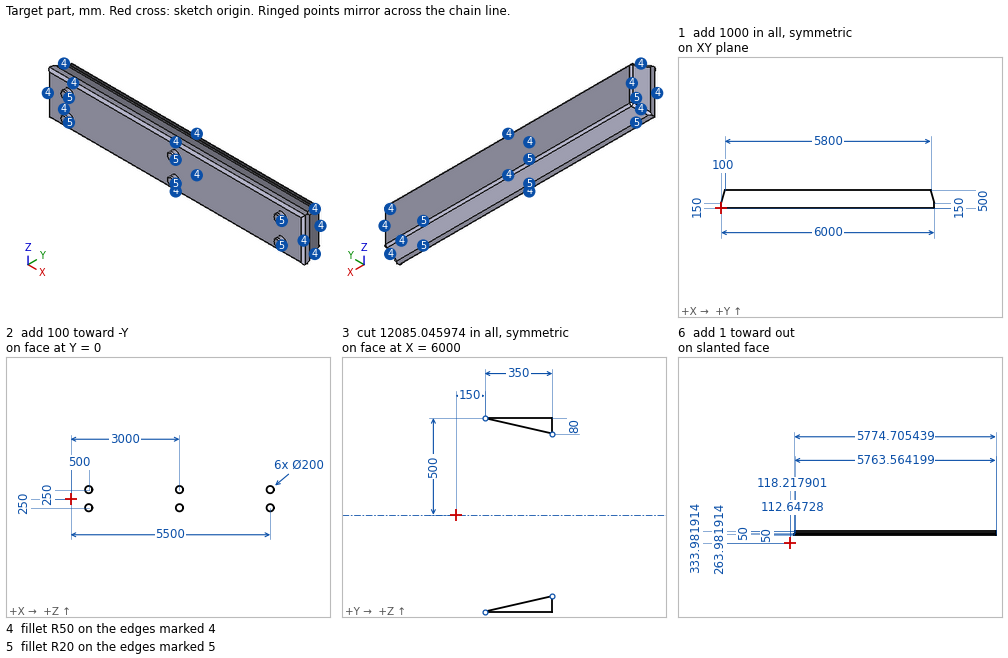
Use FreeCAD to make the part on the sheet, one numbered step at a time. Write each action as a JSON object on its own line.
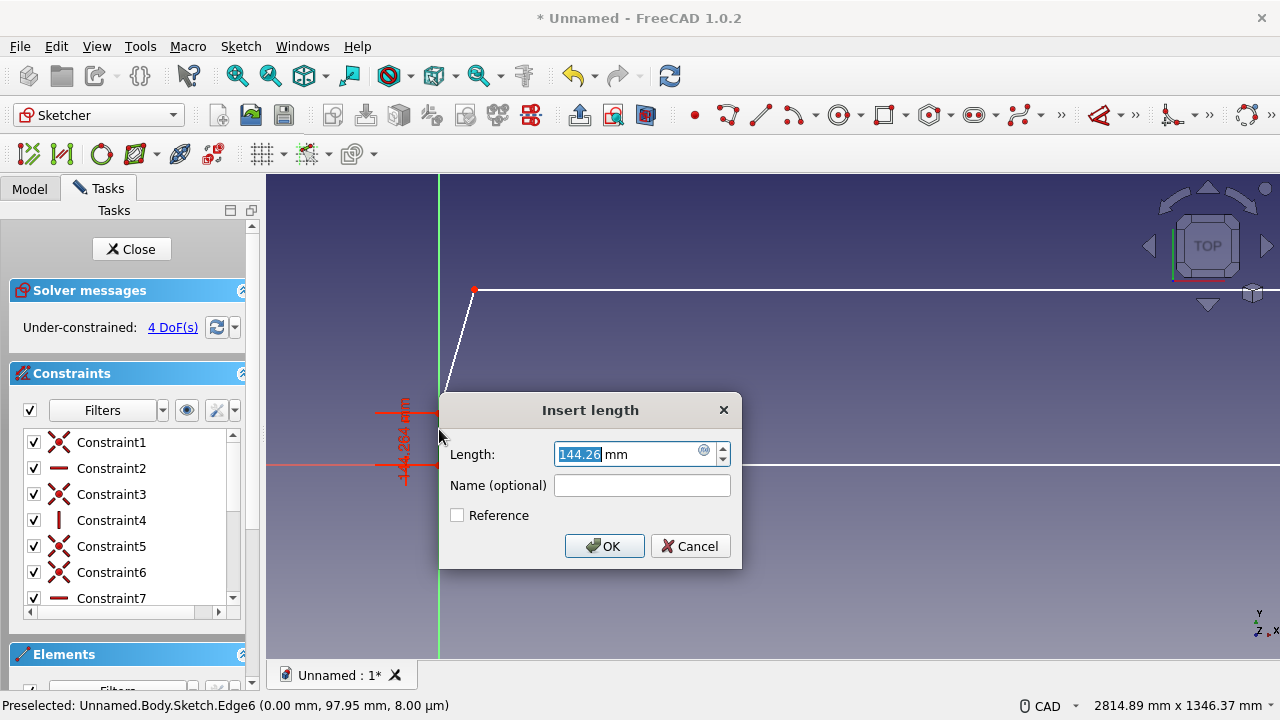
{"action": "type", "text": "150"}
{"action": "key", "text": "Return"}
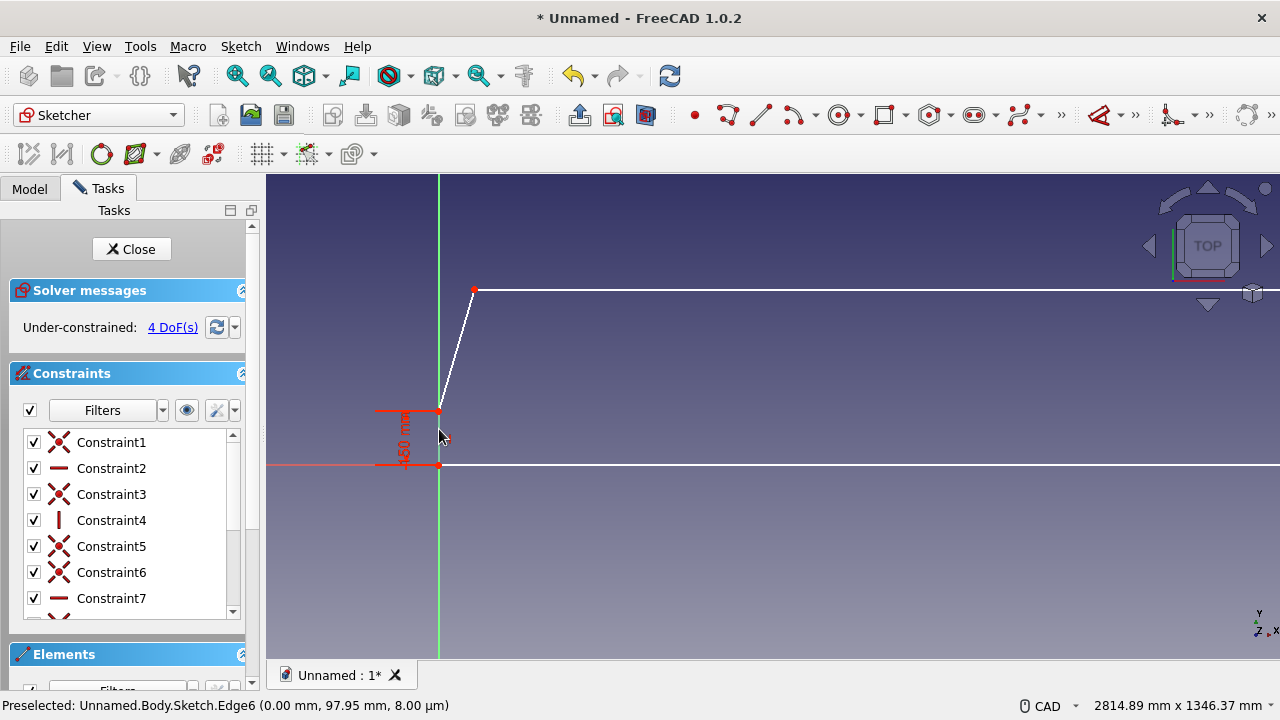
{"action": "scroll", "coordinate": [438, 430], "scroll_direction": "down", "scroll_amount": 7}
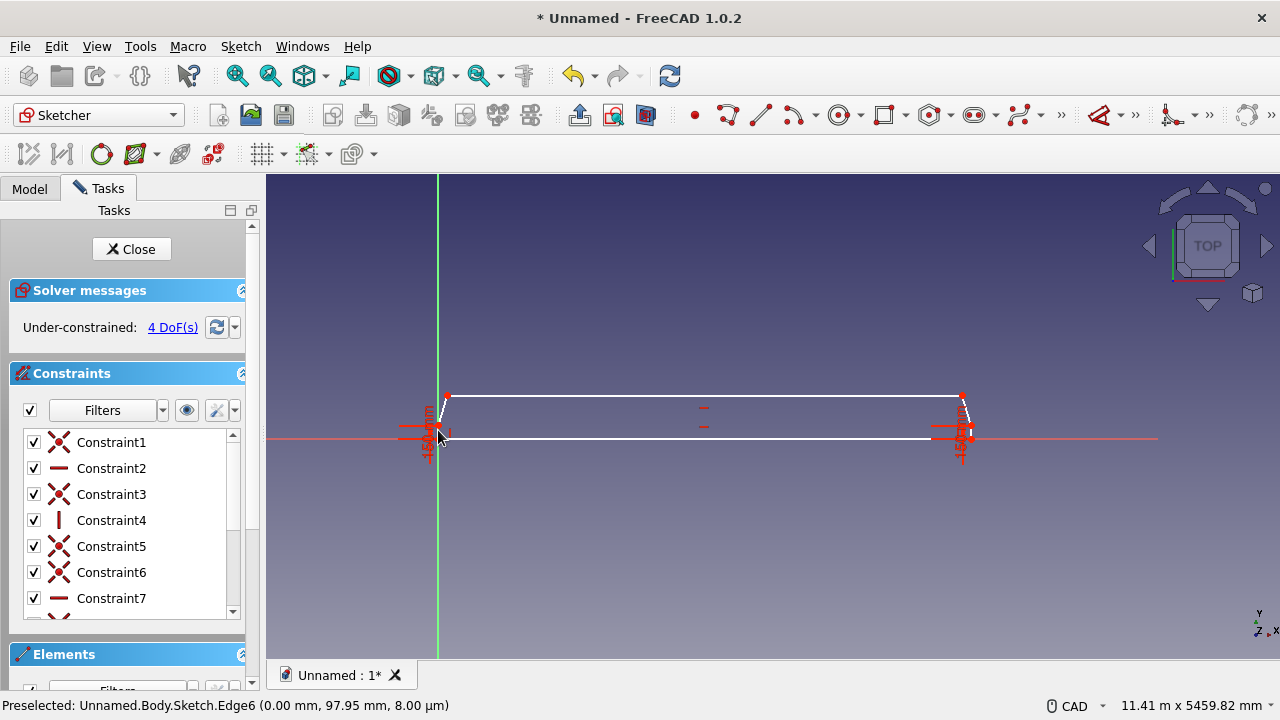
{"action": "left_click", "coordinate": [598, 439]}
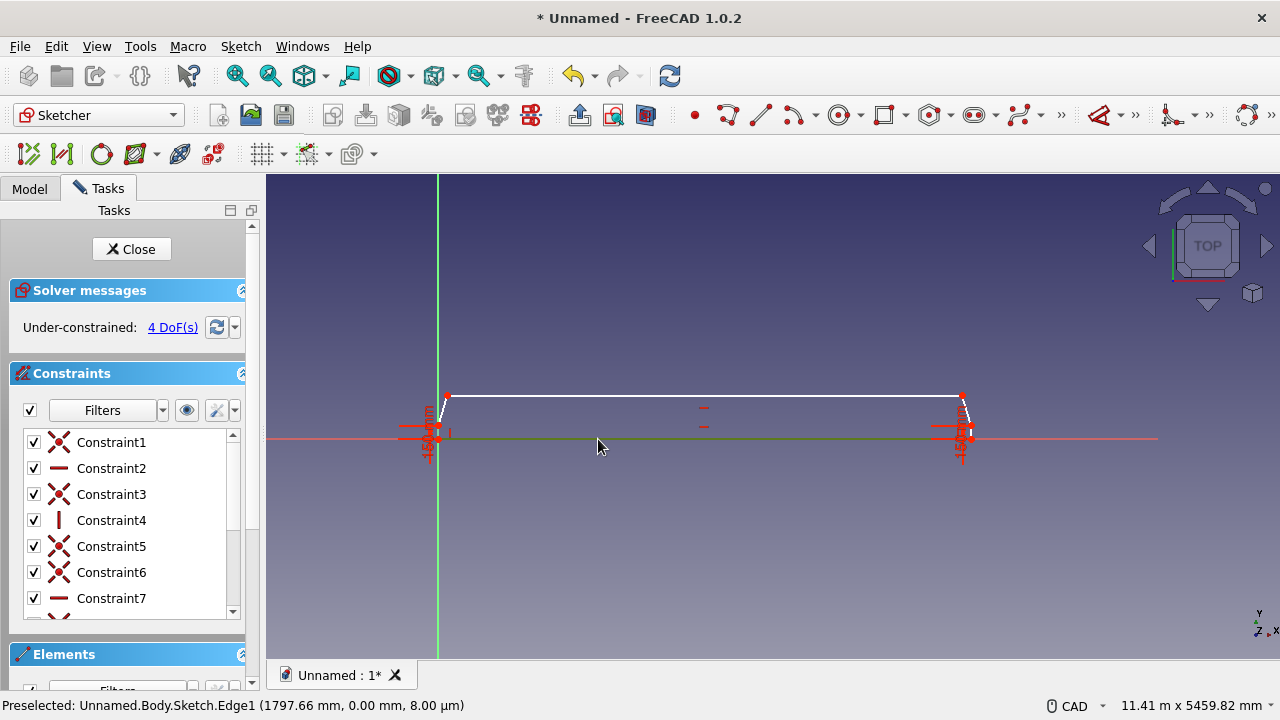
{"action": "left_click", "coordinate": [1120, 116]}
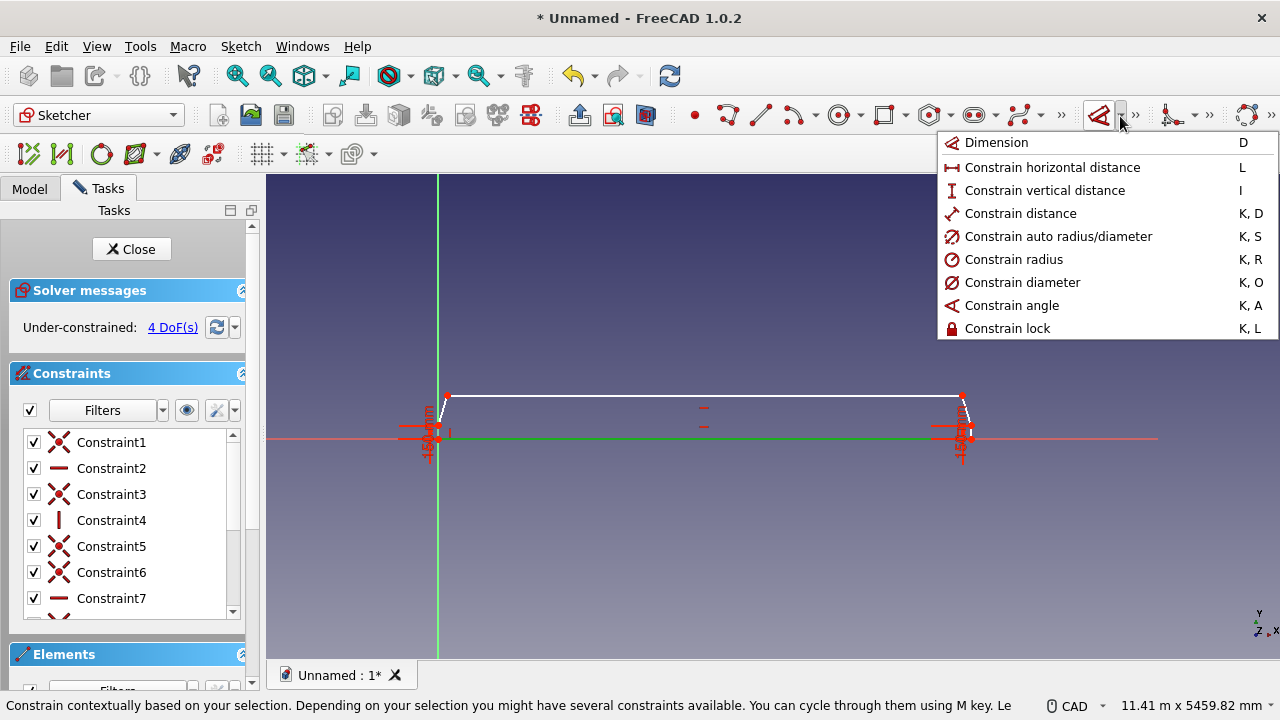
{"action": "left_click", "coordinate": [1108, 168]}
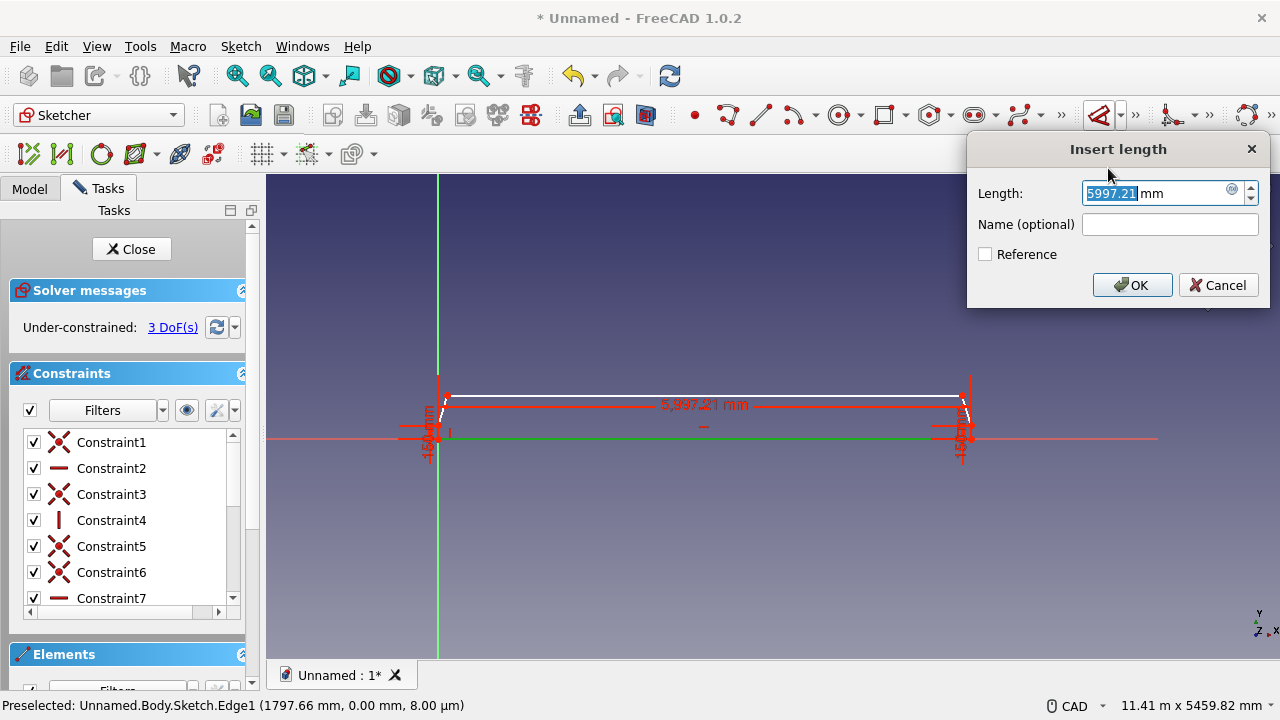
{"action": "type", "text": "6000"}
{"action": "key", "text": "Return"}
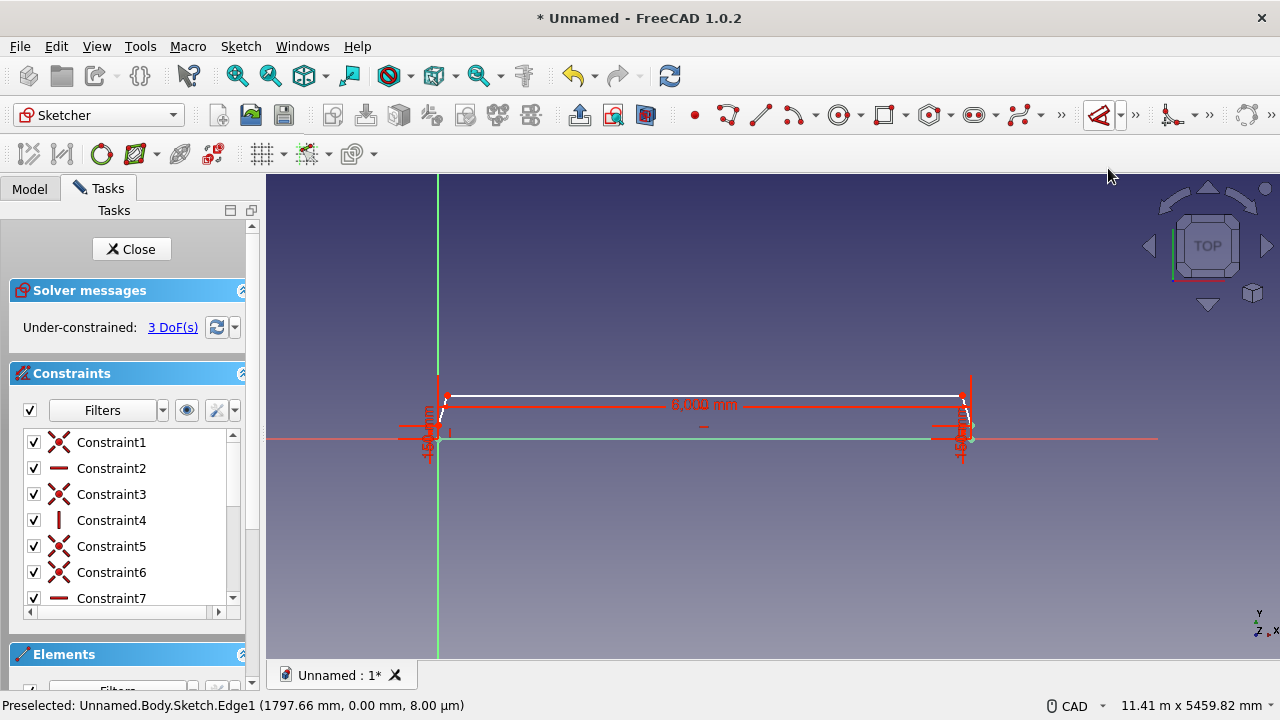
{"action": "left_click", "coordinate": [808, 396]}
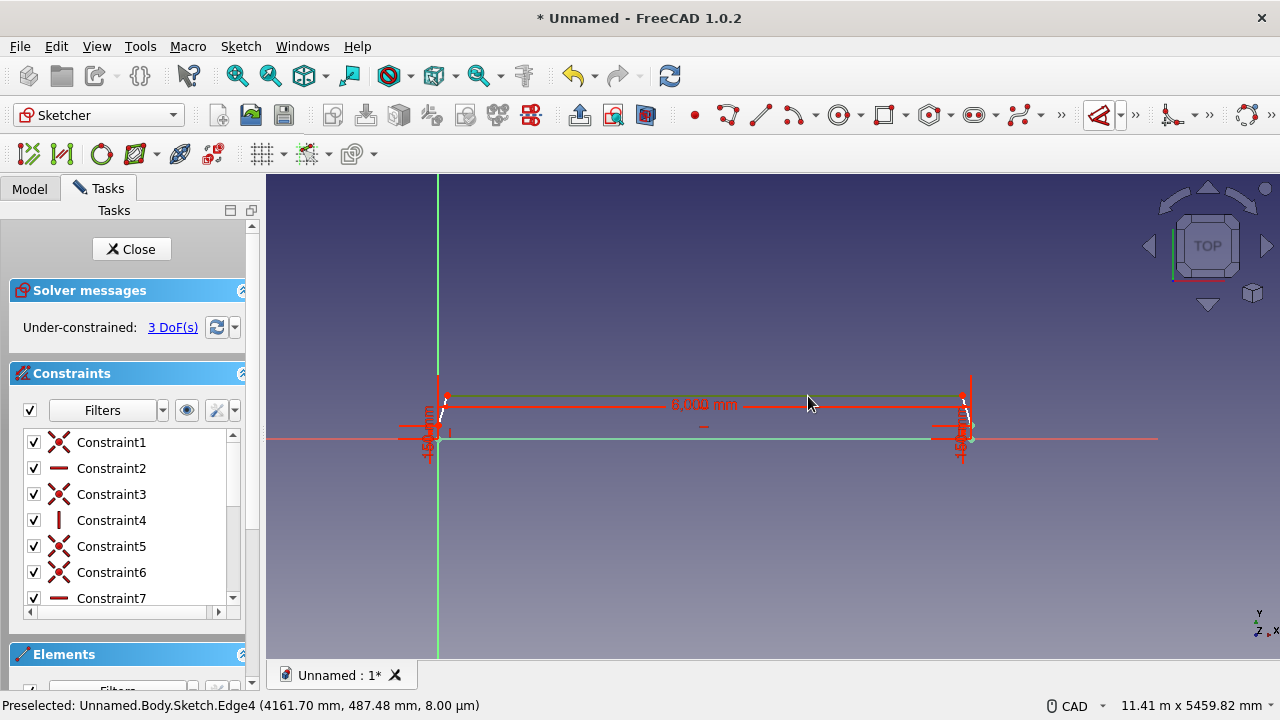
{"action": "left_click", "coordinate": [1120, 116]}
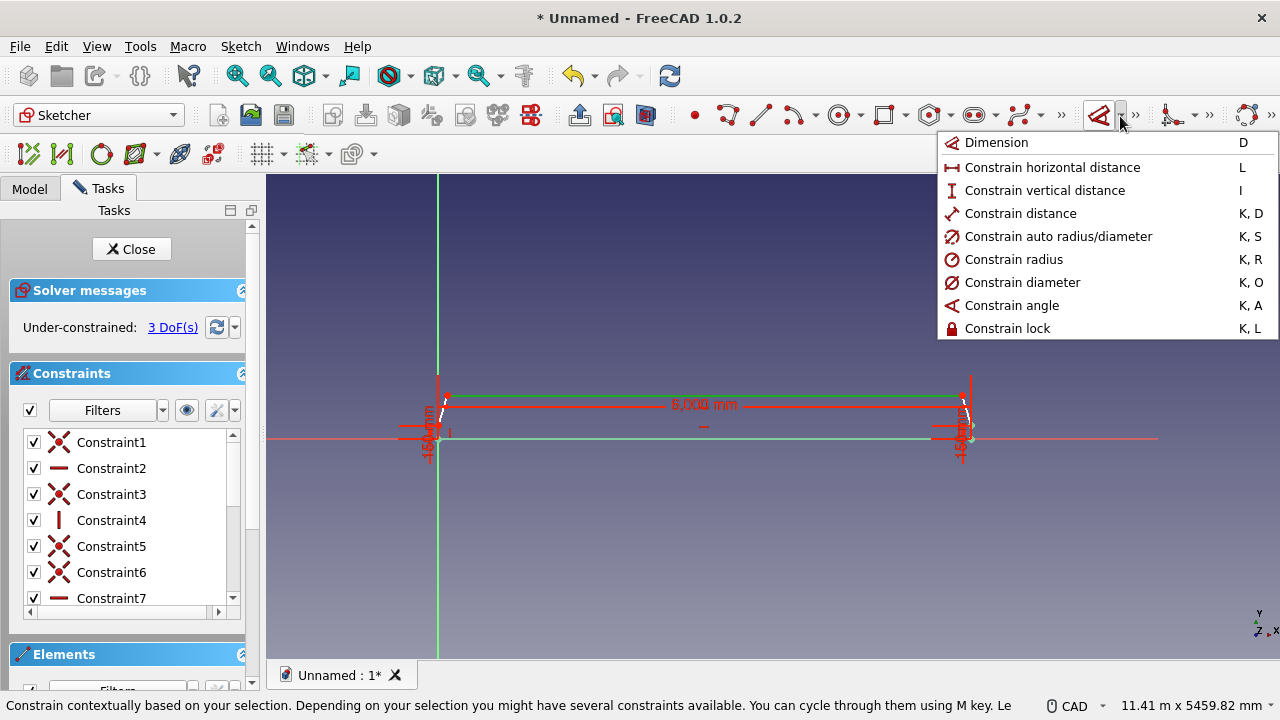
{"action": "left_click", "coordinate": [1108, 168]}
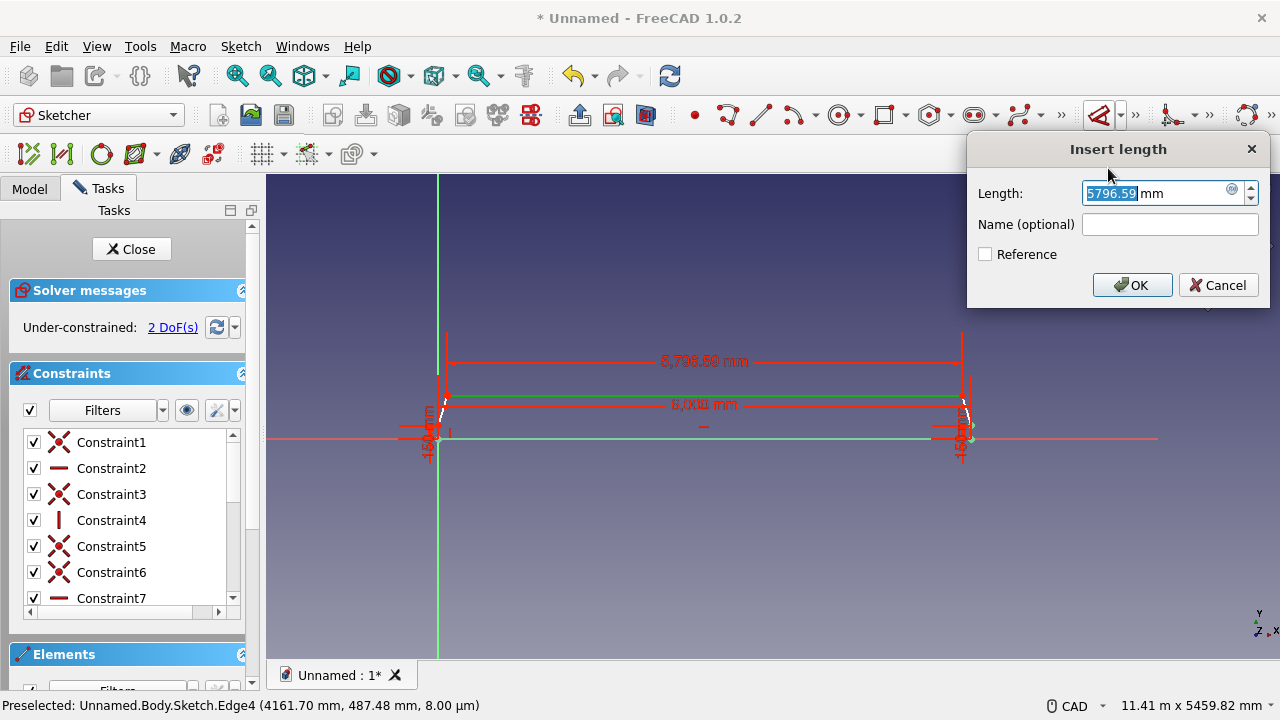
{"action": "type", "text": "5800"}
{"action": "key", "text": "Return"}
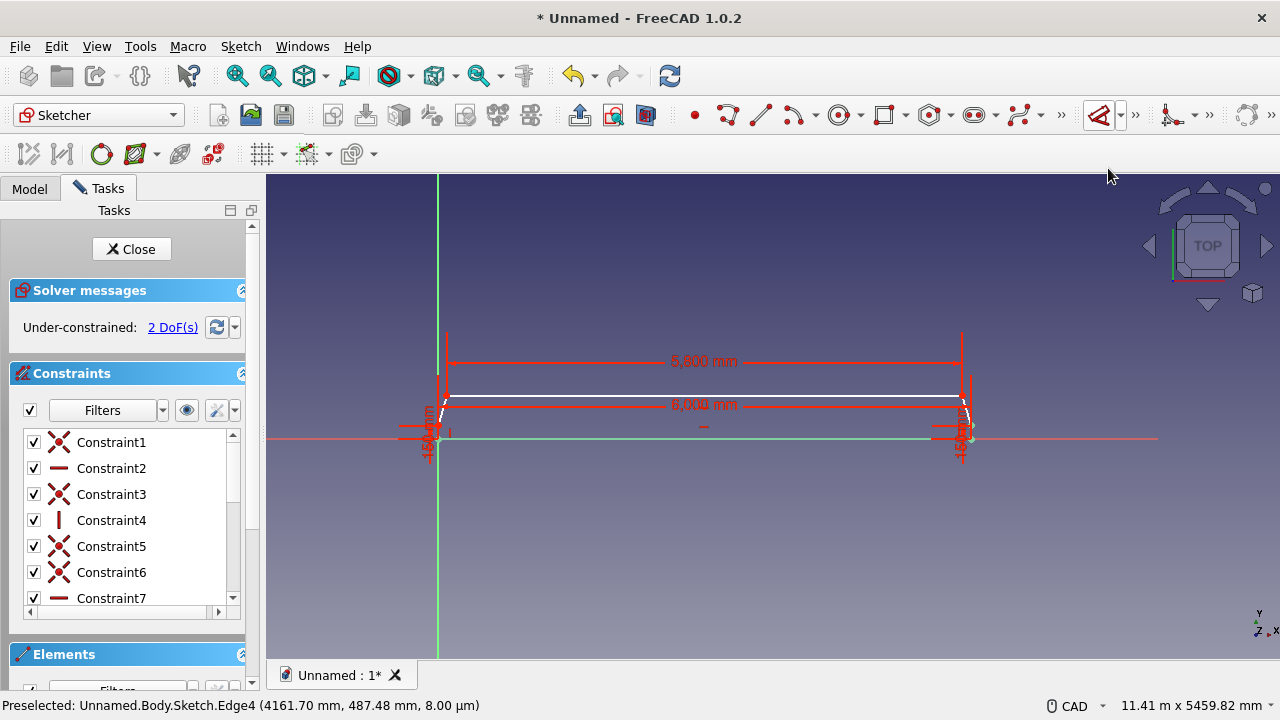
{"action": "left_click", "coordinate": [962, 396]}